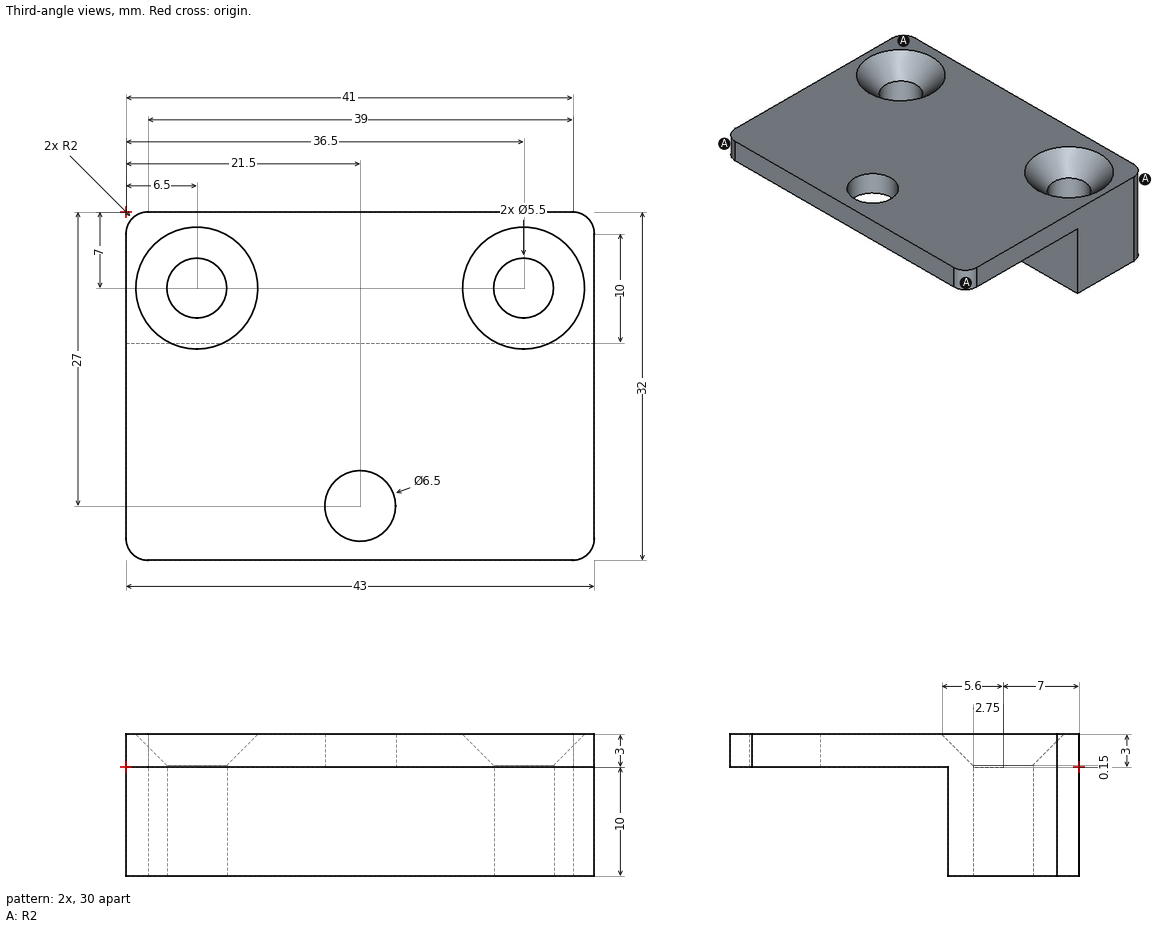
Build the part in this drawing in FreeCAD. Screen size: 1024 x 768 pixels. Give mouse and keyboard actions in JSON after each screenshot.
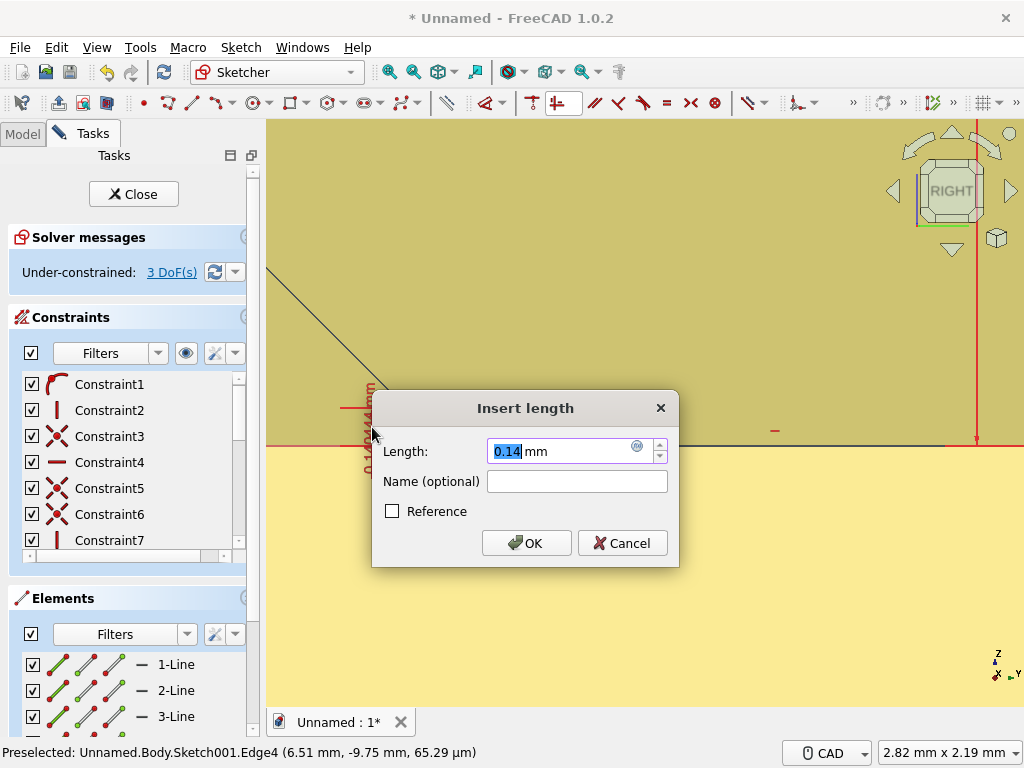
{"action": "type", "text": "0.15"}
{"action": "key", "text": "Return"}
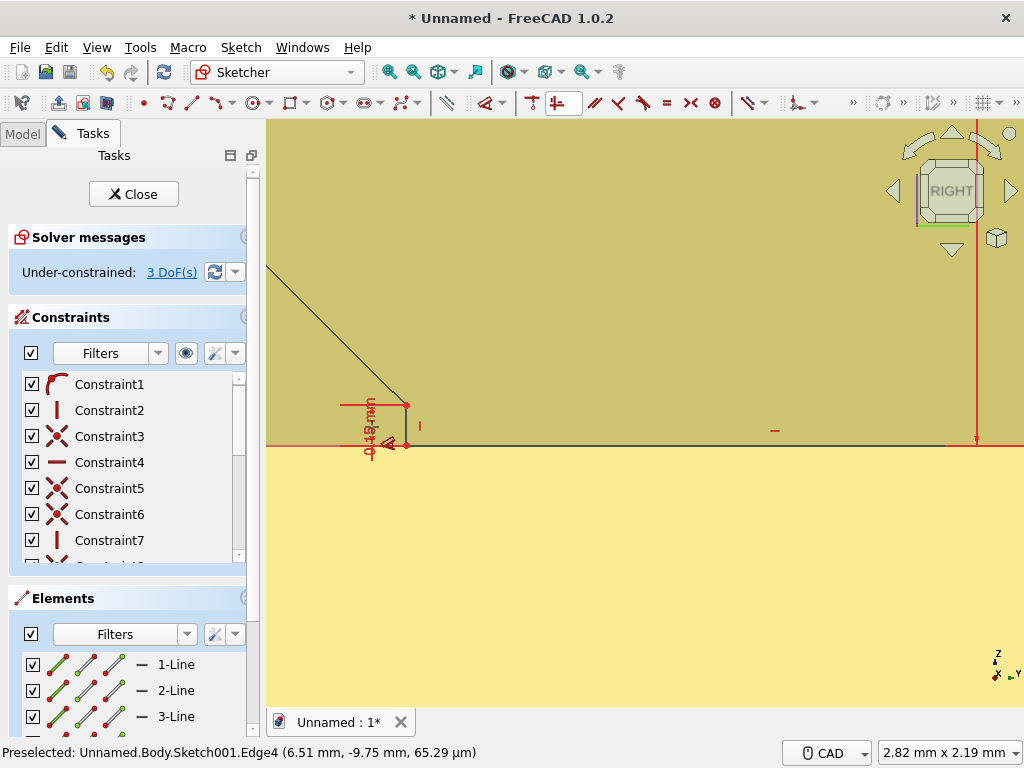
{"action": "scroll", "coordinate": [482, 439], "scroll_direction": "down", "scroll_amount": 11}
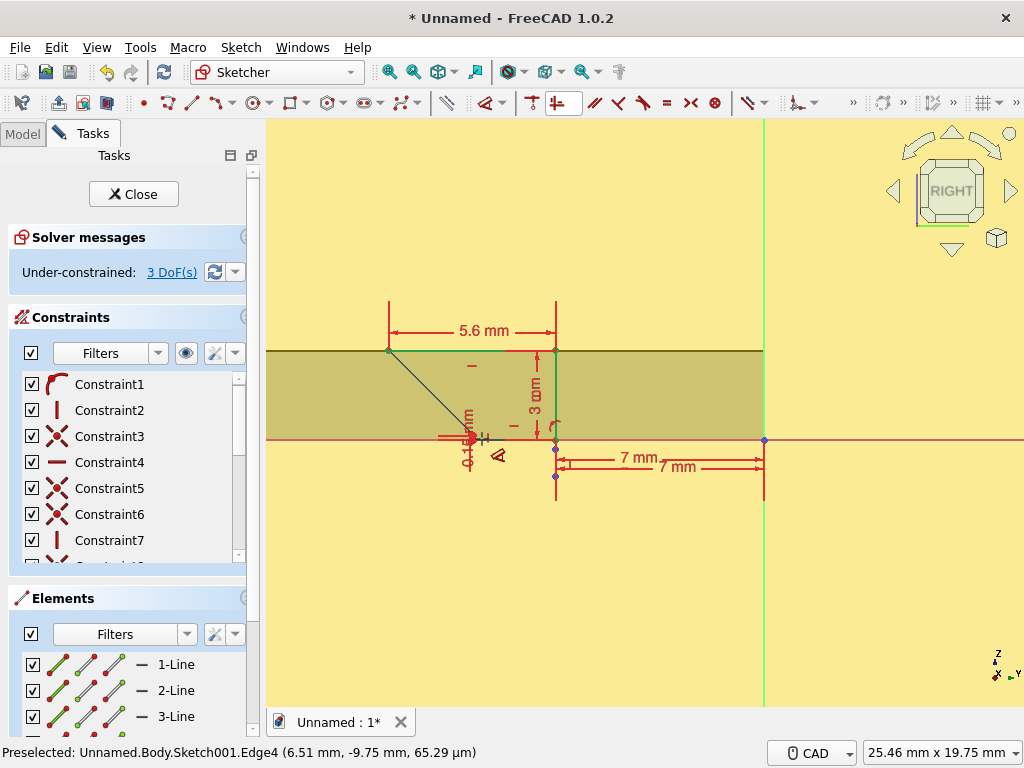
{"action": "left_click", "coordinate": [498, 440]}
{"action": "left_click", "coordinate": [515, 474]}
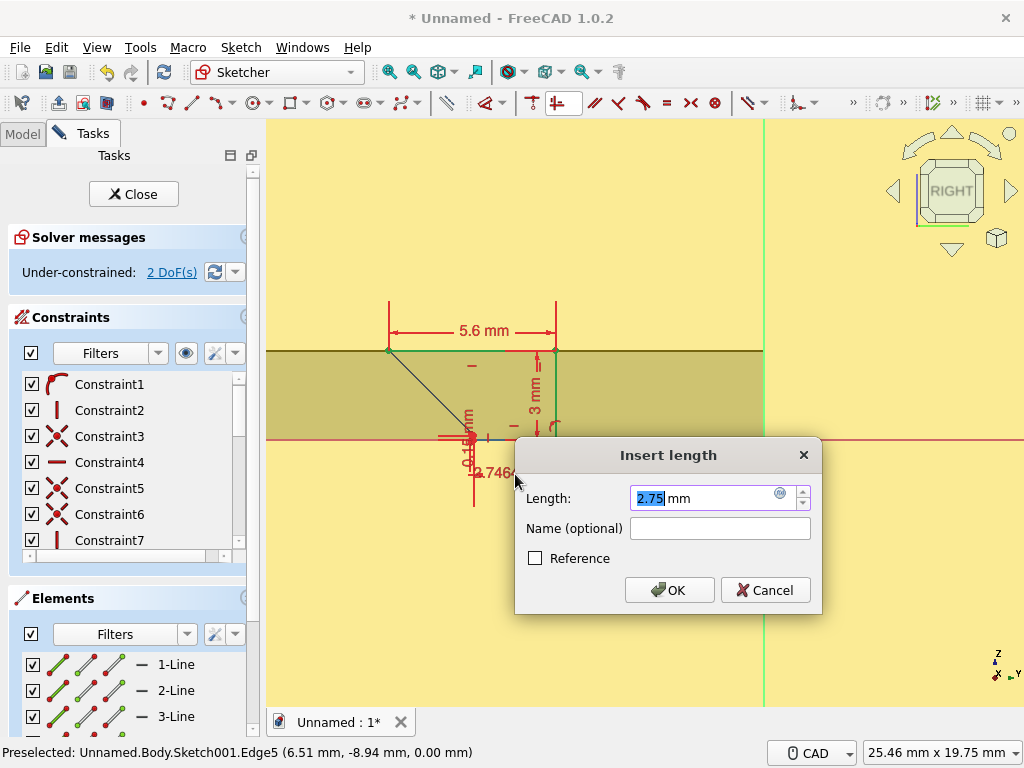
{"action": "type", "text": "2.75"}
{"action": "key", "text": "Return"}
{"action": "key", "text": "Escape"}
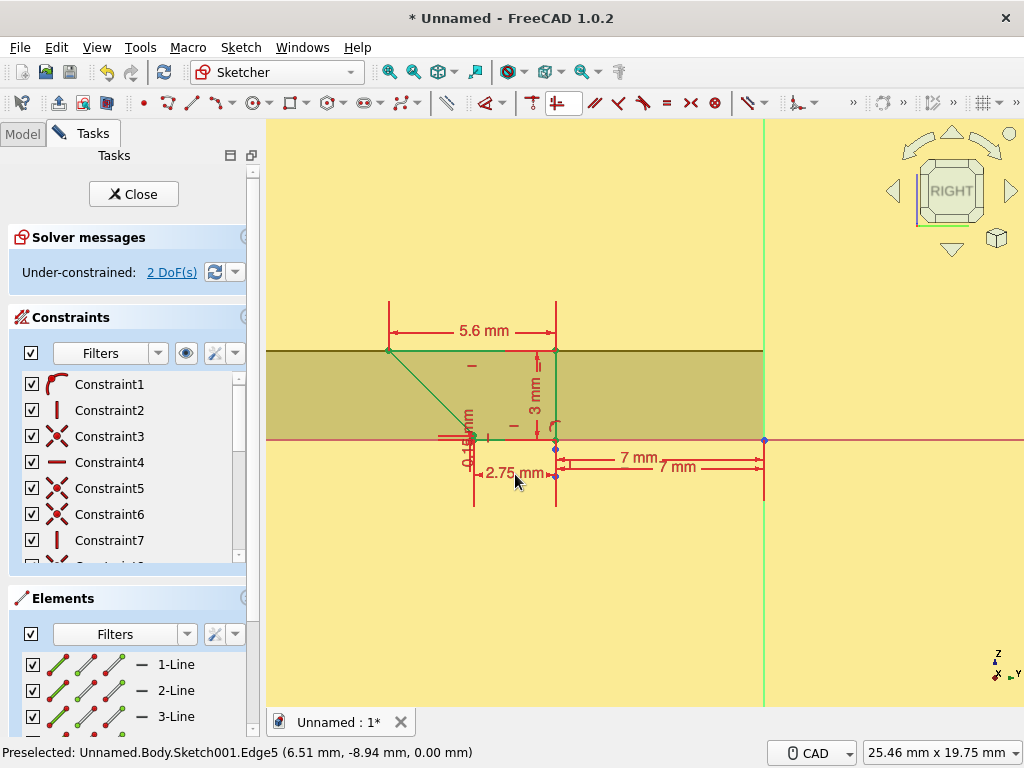
{"action": "left_click", "coordinate": [134, 194]}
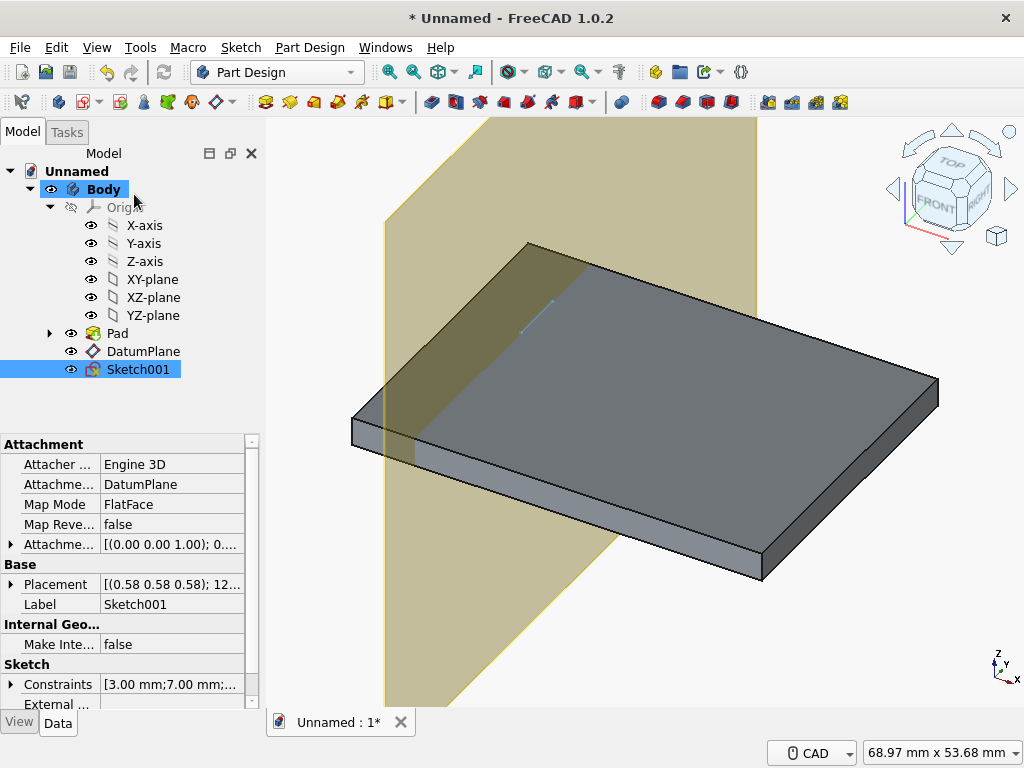
{"action": "left_click", "coordinate": [480, 102]}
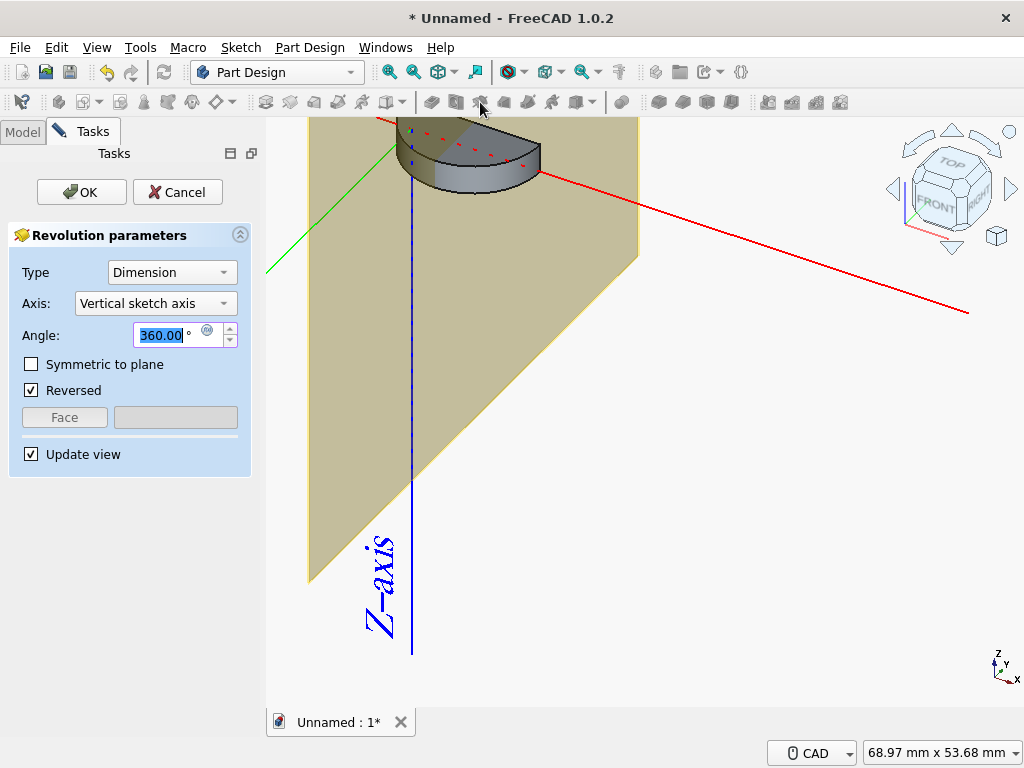
{"action": "left_click", "coordinate": [156, 304]}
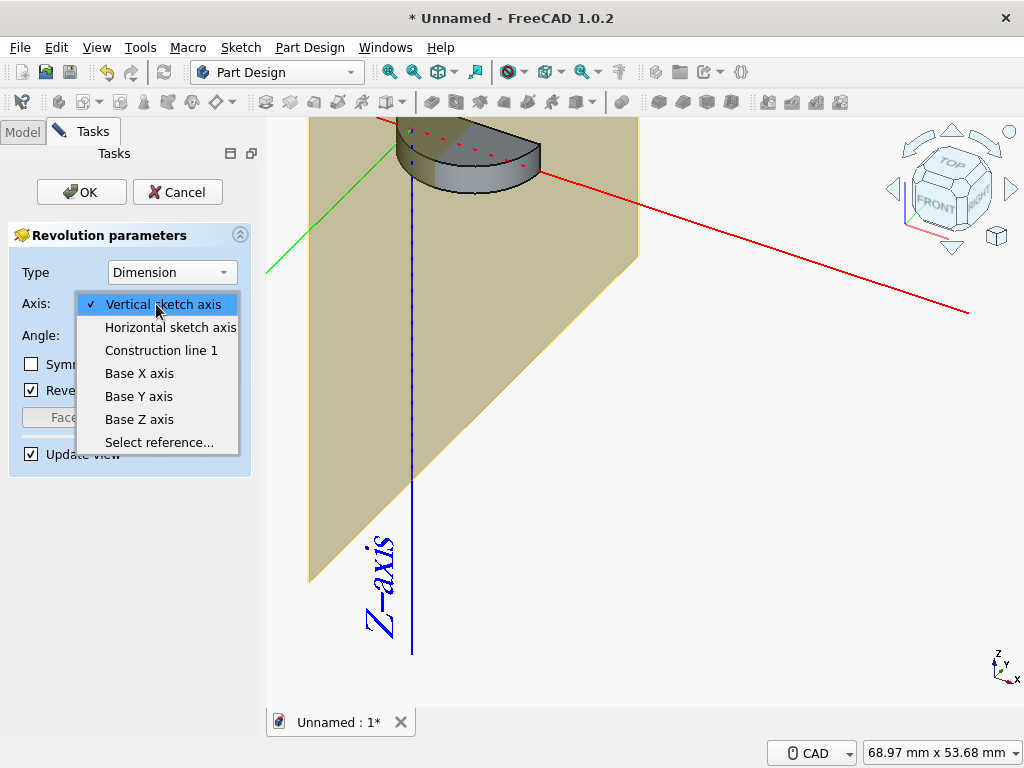
{"action": "left_click", "coordinate": [156, 350]}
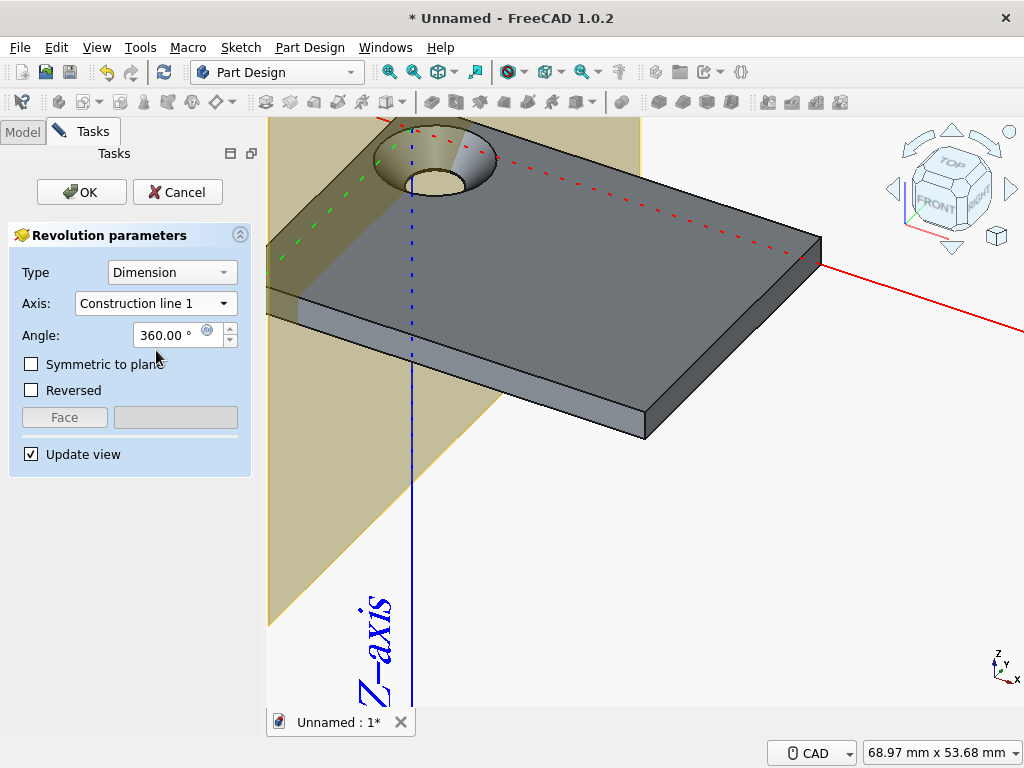
{"action": "left_click", "coordinate": [82, 192]}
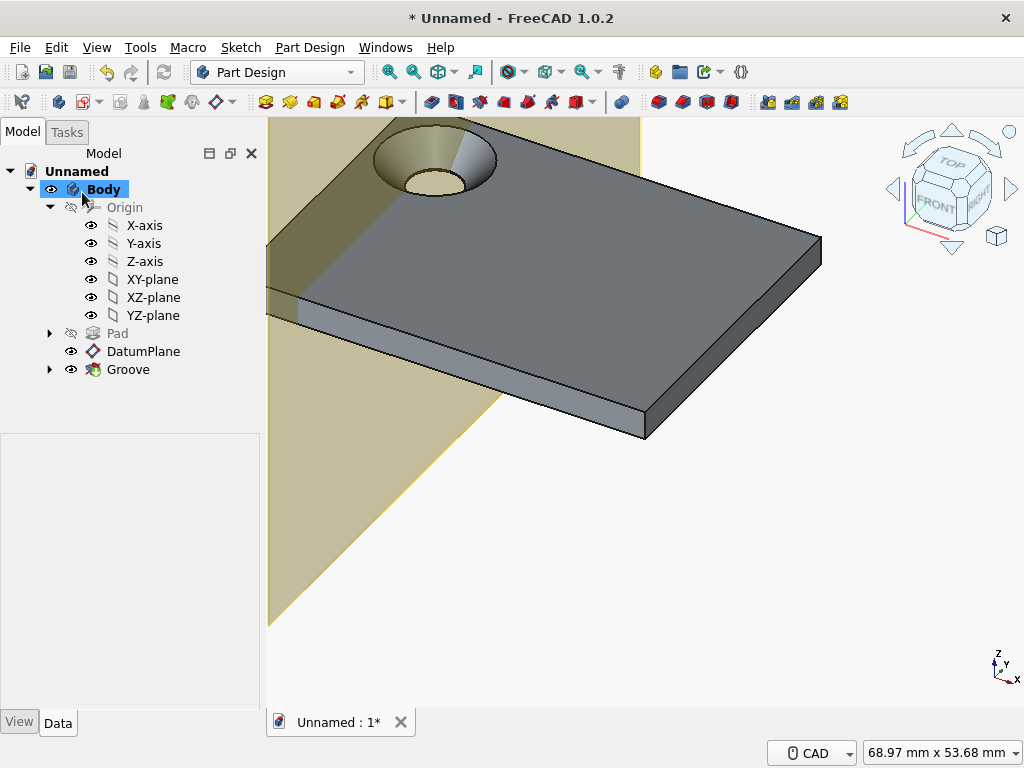
{"action": "left_click", "coordinate": [116, 351]}
{"action": "key", "text": "space"}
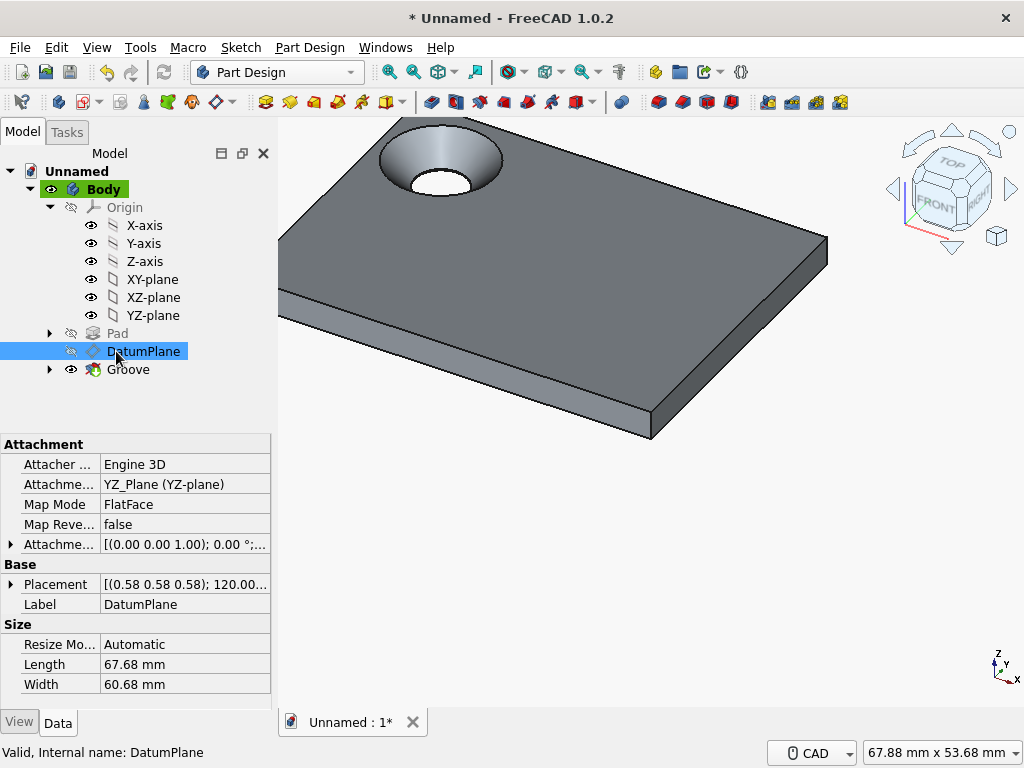
{"action": "left_click", "coordinate": [390, 72]}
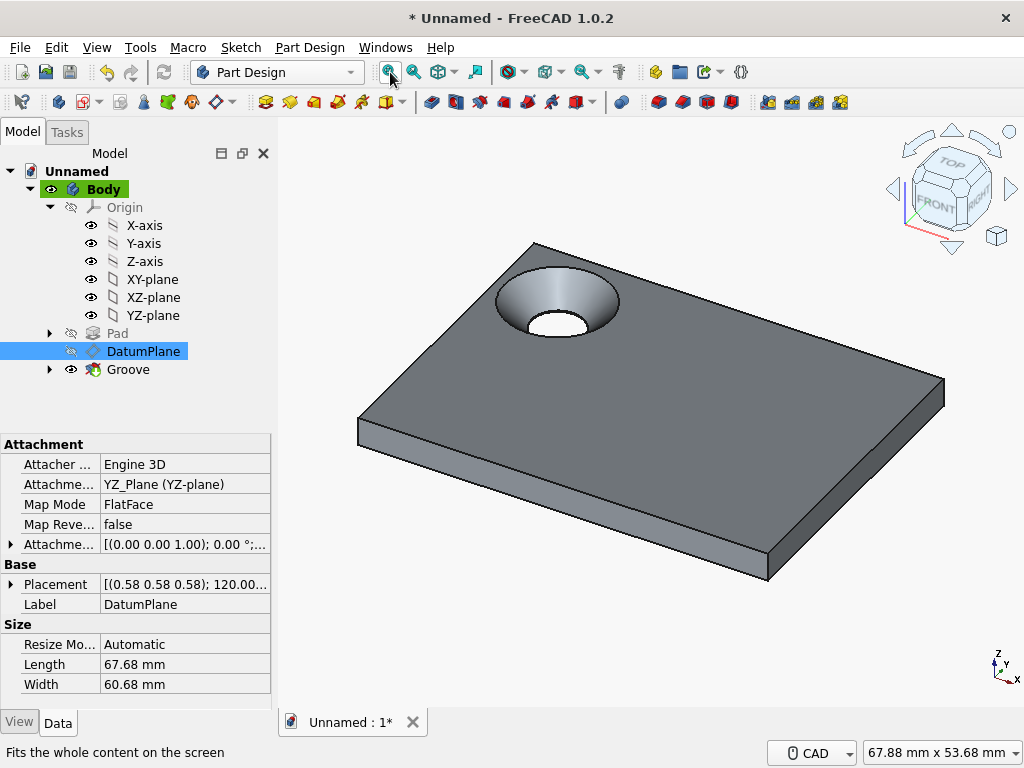
{"action": "left_click", "coordinate": [116, 369]}